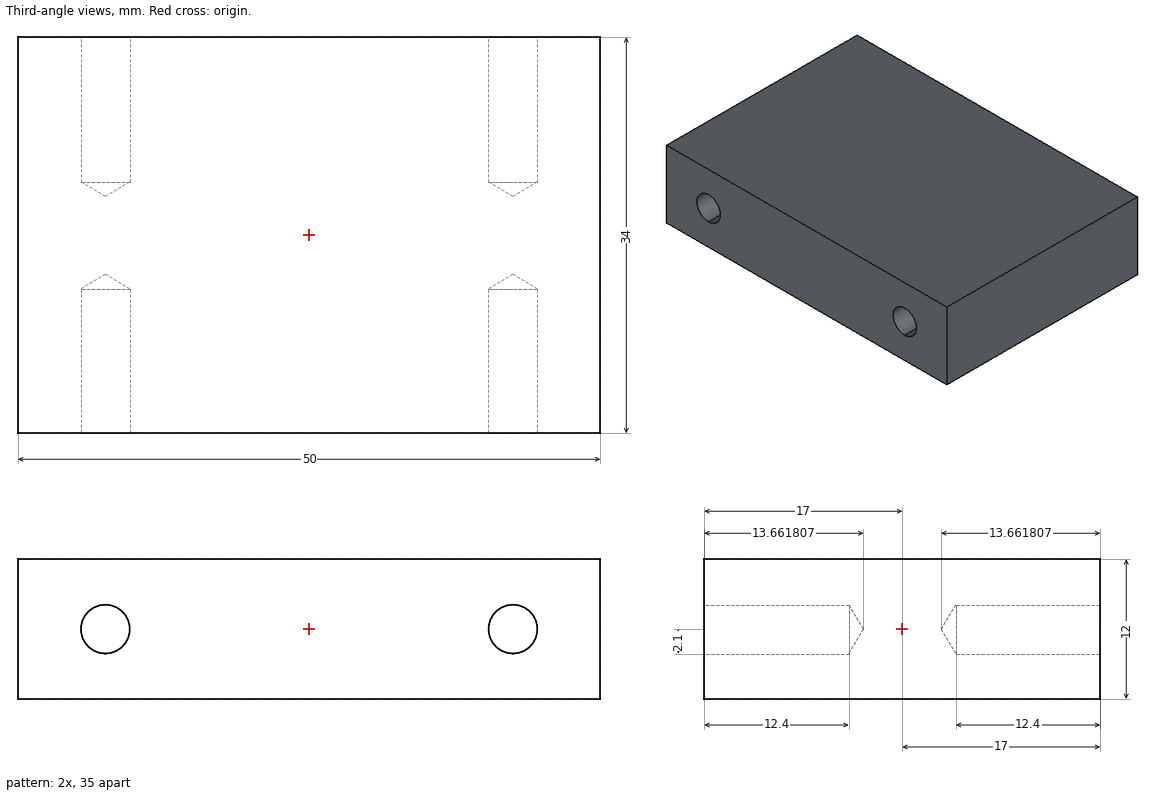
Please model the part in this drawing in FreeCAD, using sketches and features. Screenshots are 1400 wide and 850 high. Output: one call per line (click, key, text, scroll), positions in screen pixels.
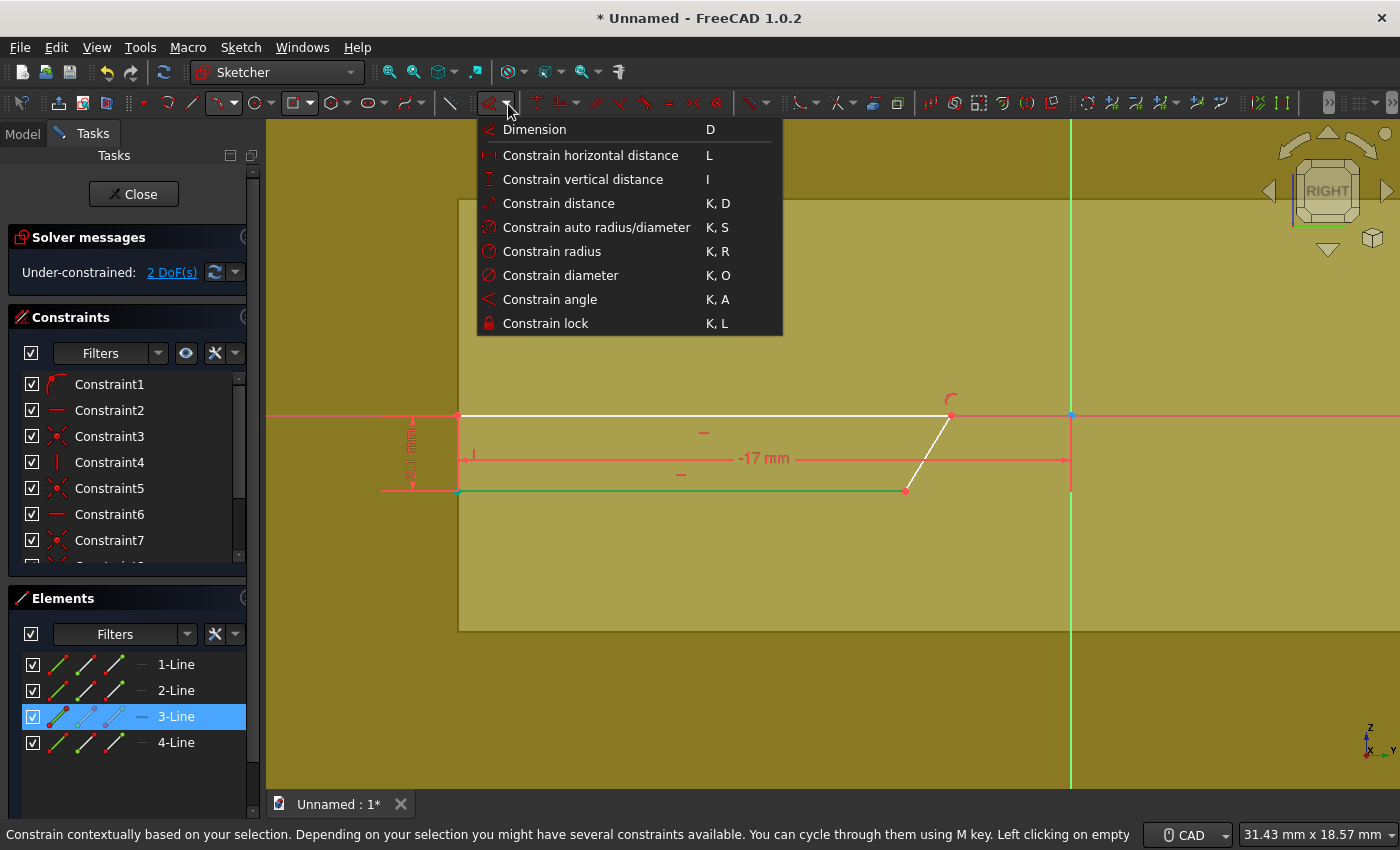
click(630, 155)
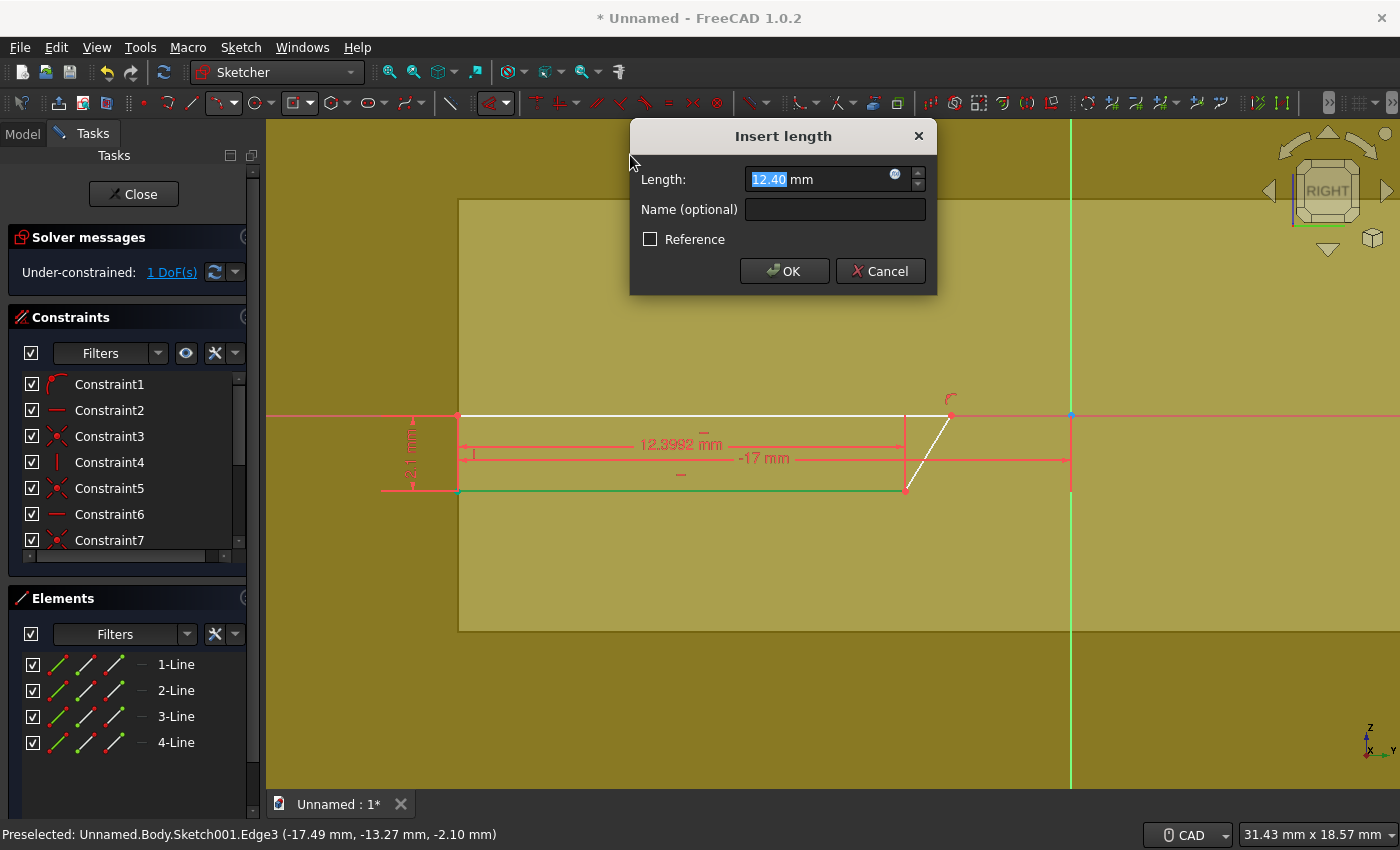
text(12.4)
key(Return)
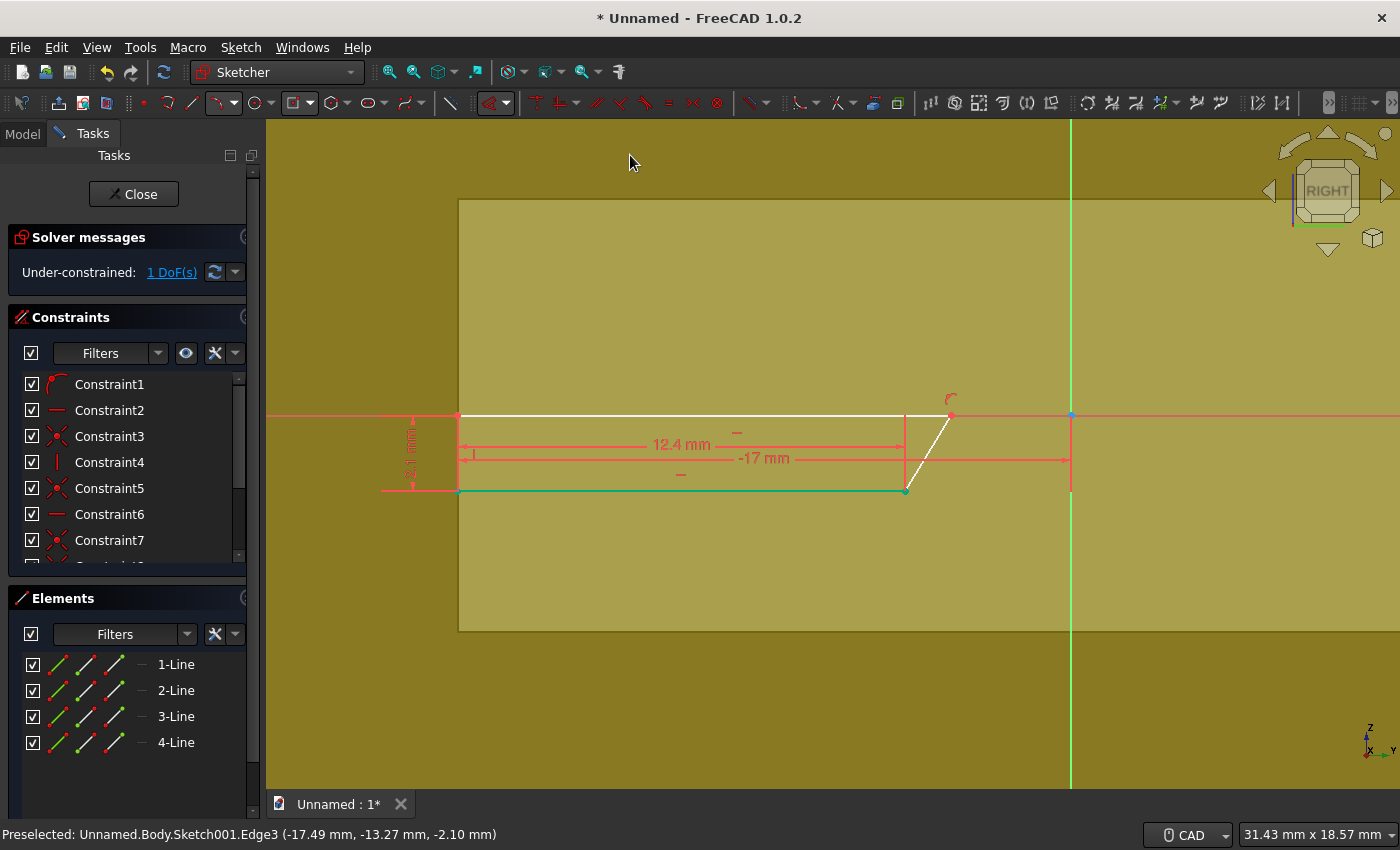
click(803, 416)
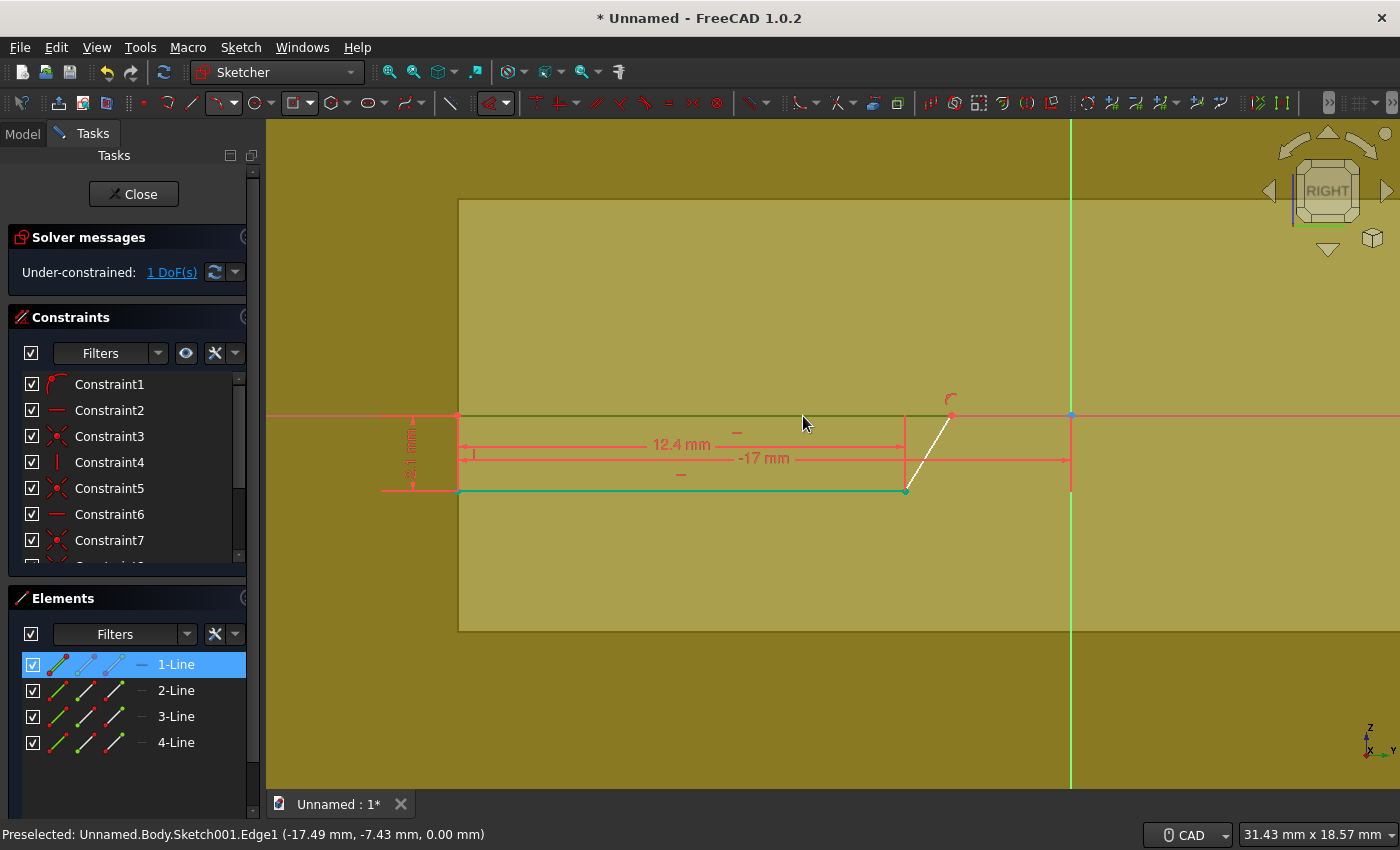
key(l)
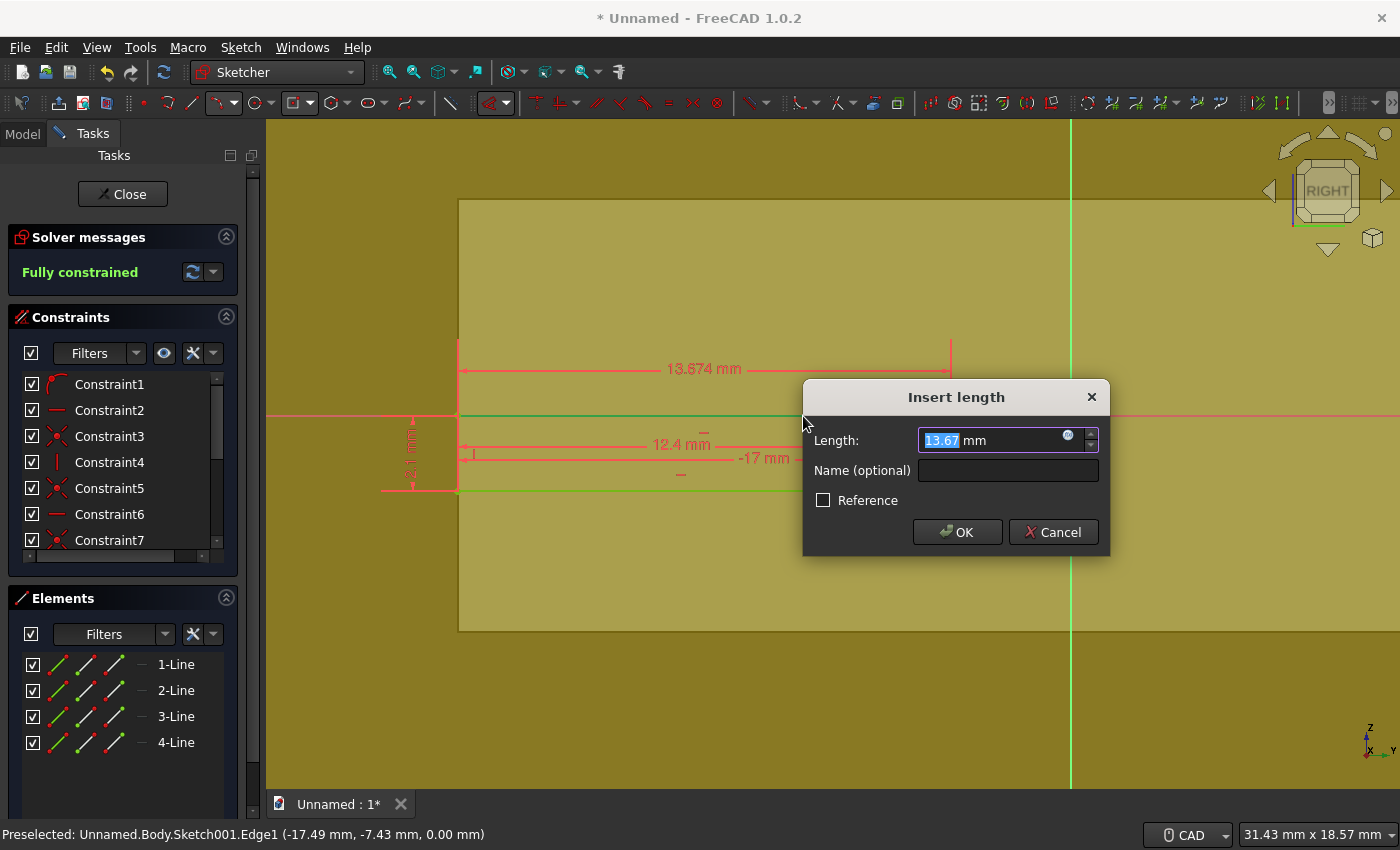
text(13.661807)
key(Return)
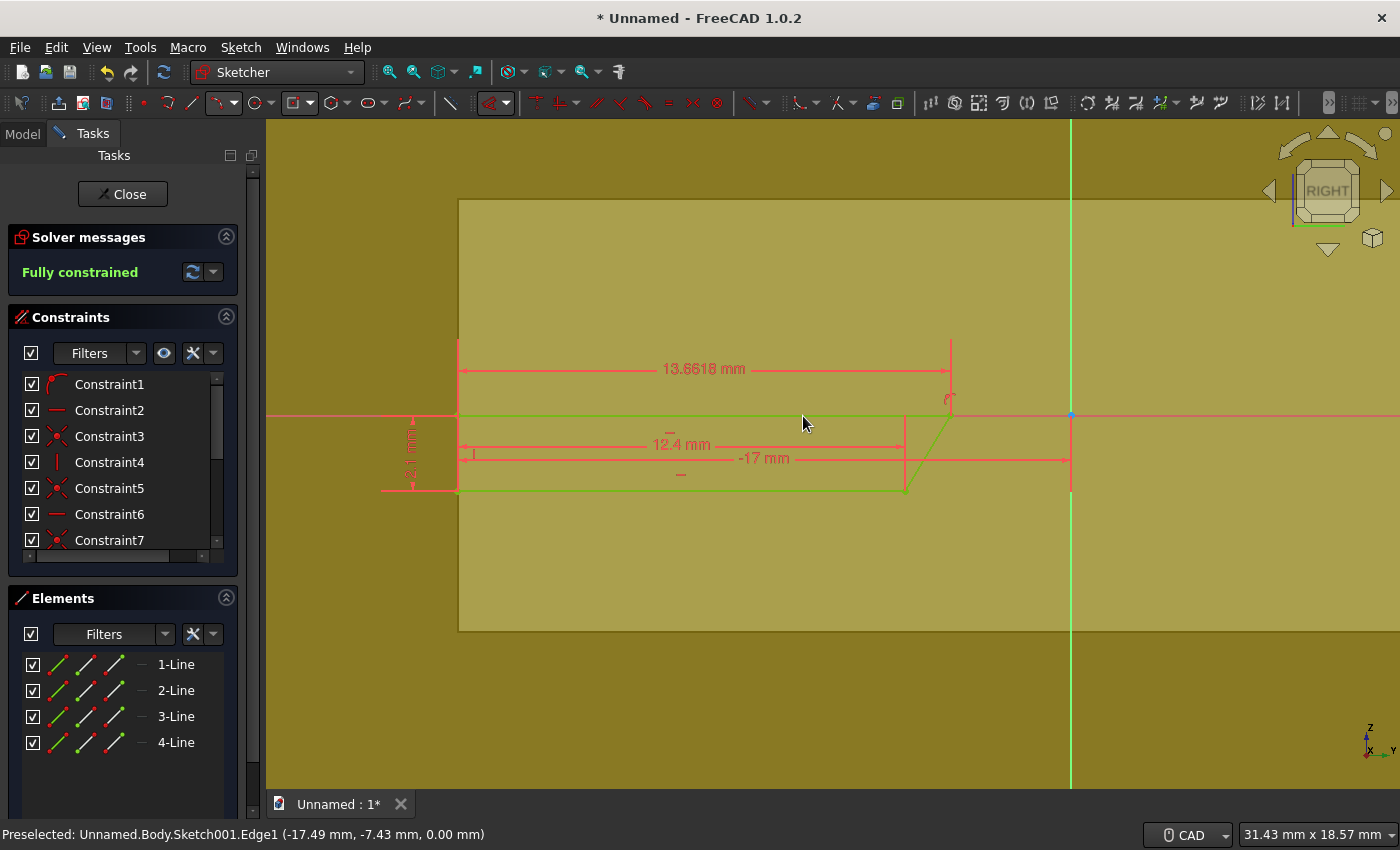
click(123, 194)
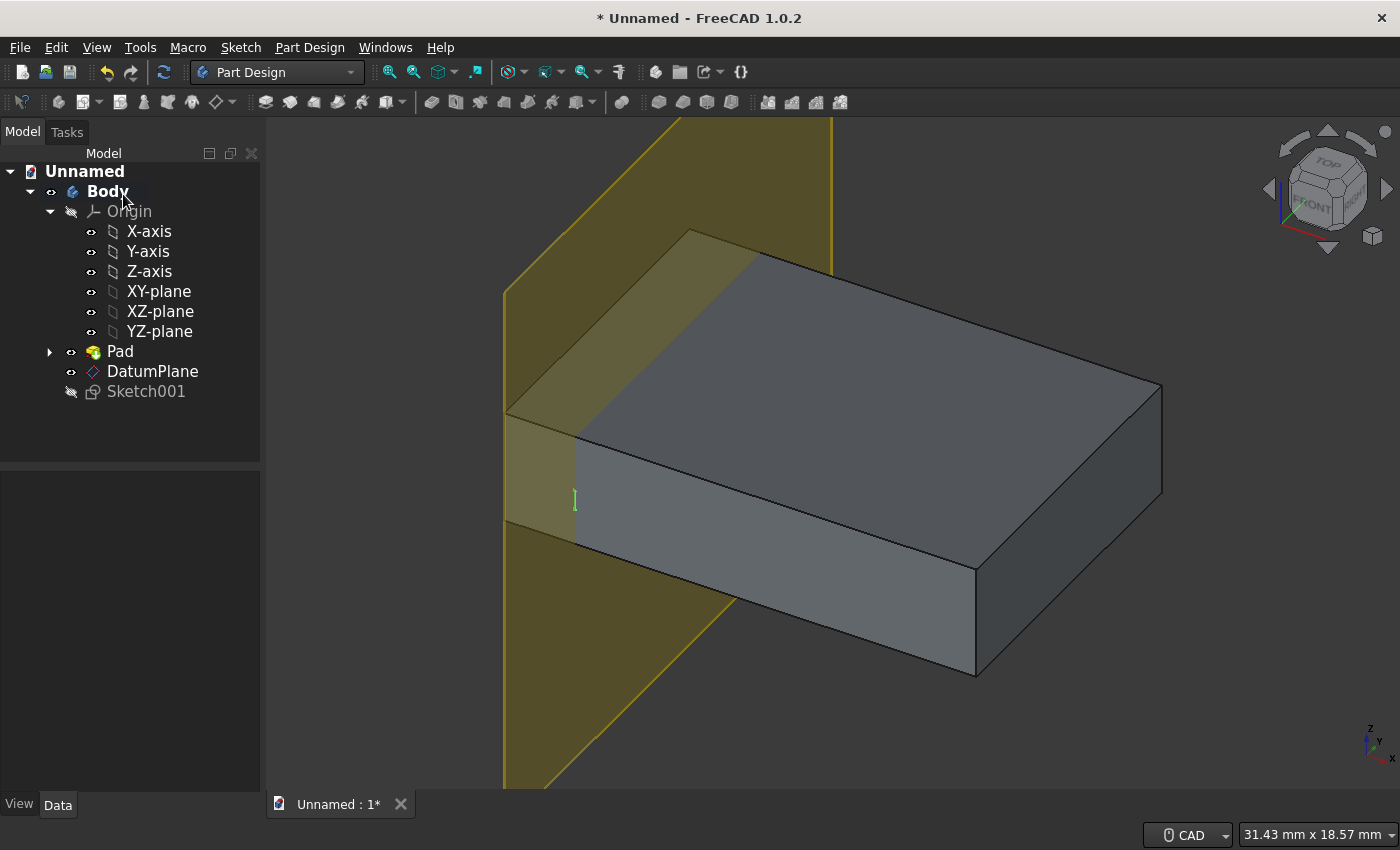
click(480, 102)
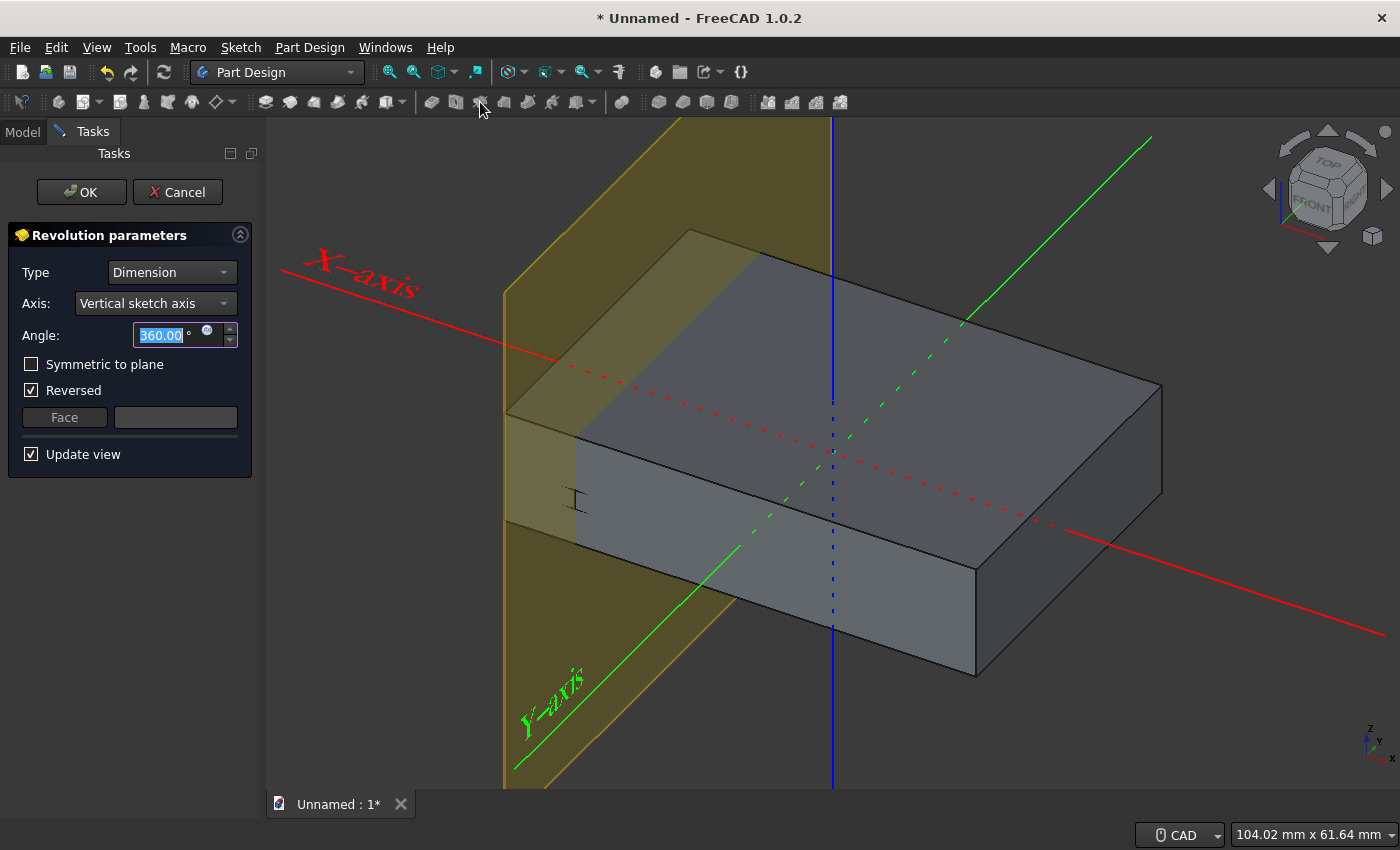
click(156, 304)